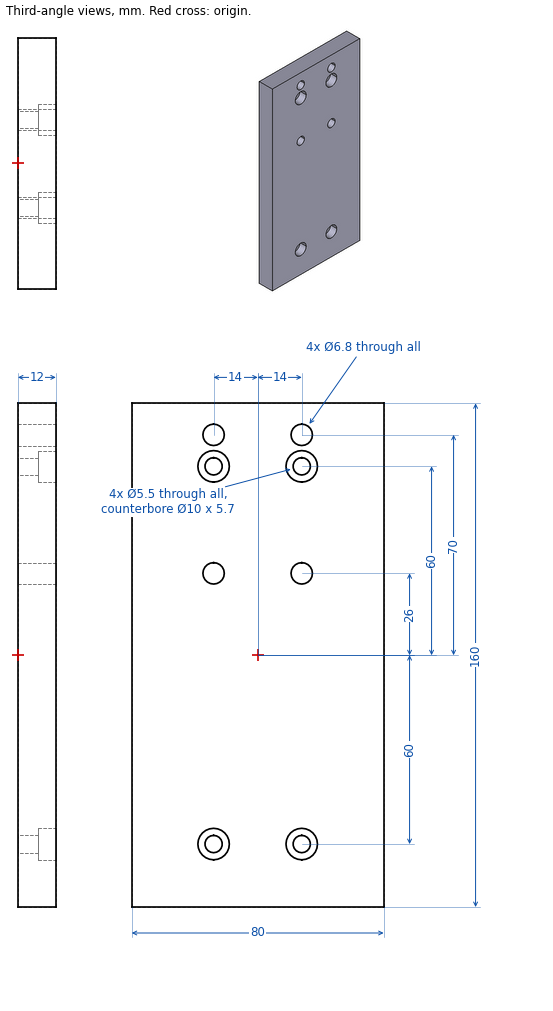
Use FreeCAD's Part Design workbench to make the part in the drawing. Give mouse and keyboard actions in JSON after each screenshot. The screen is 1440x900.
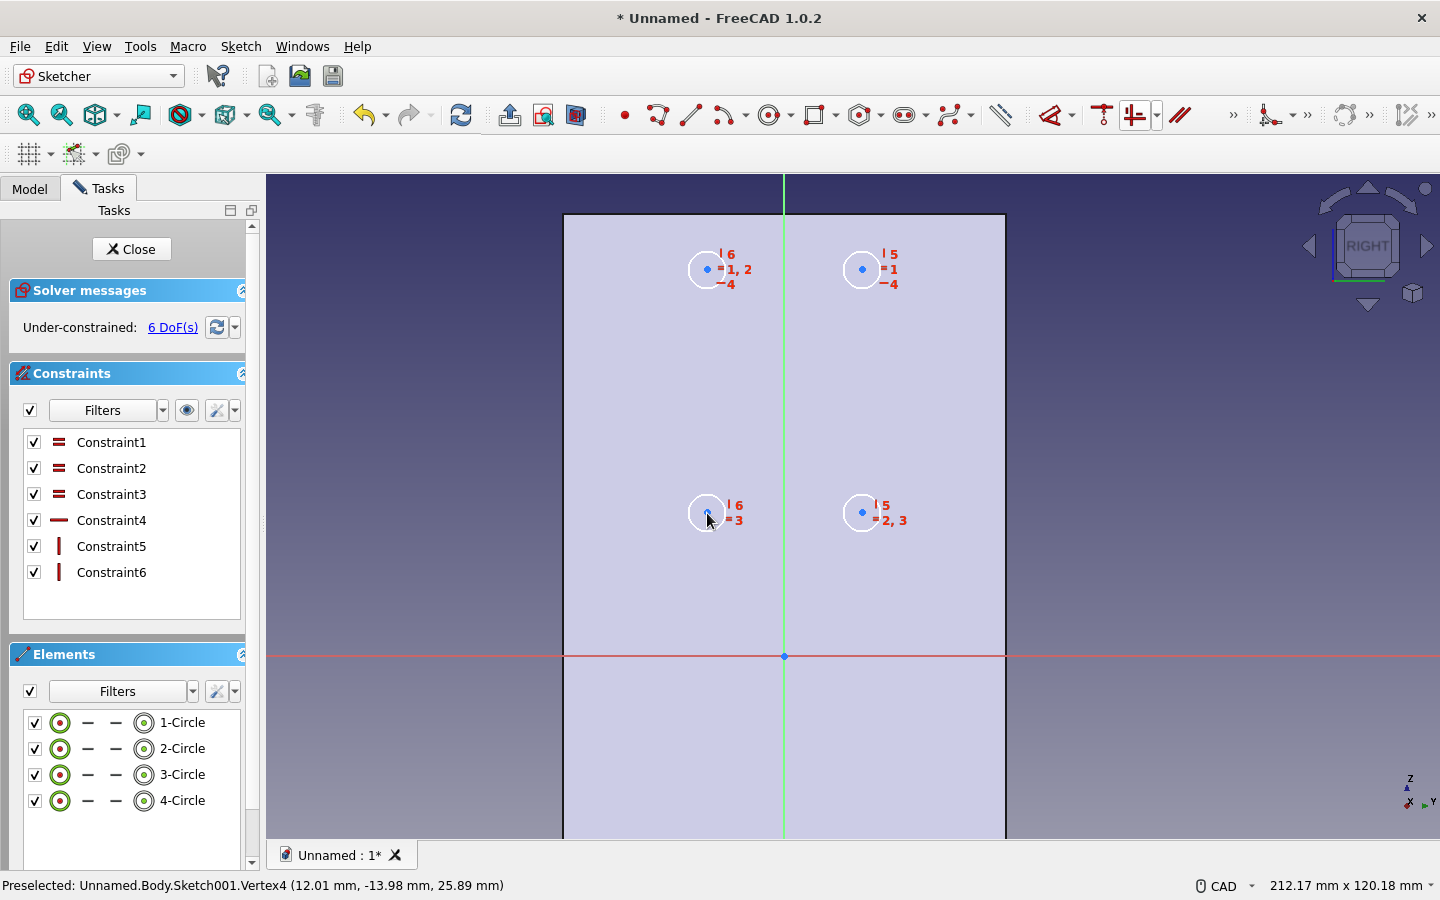
{"action": "left_click", "coordinate": [862, 513]}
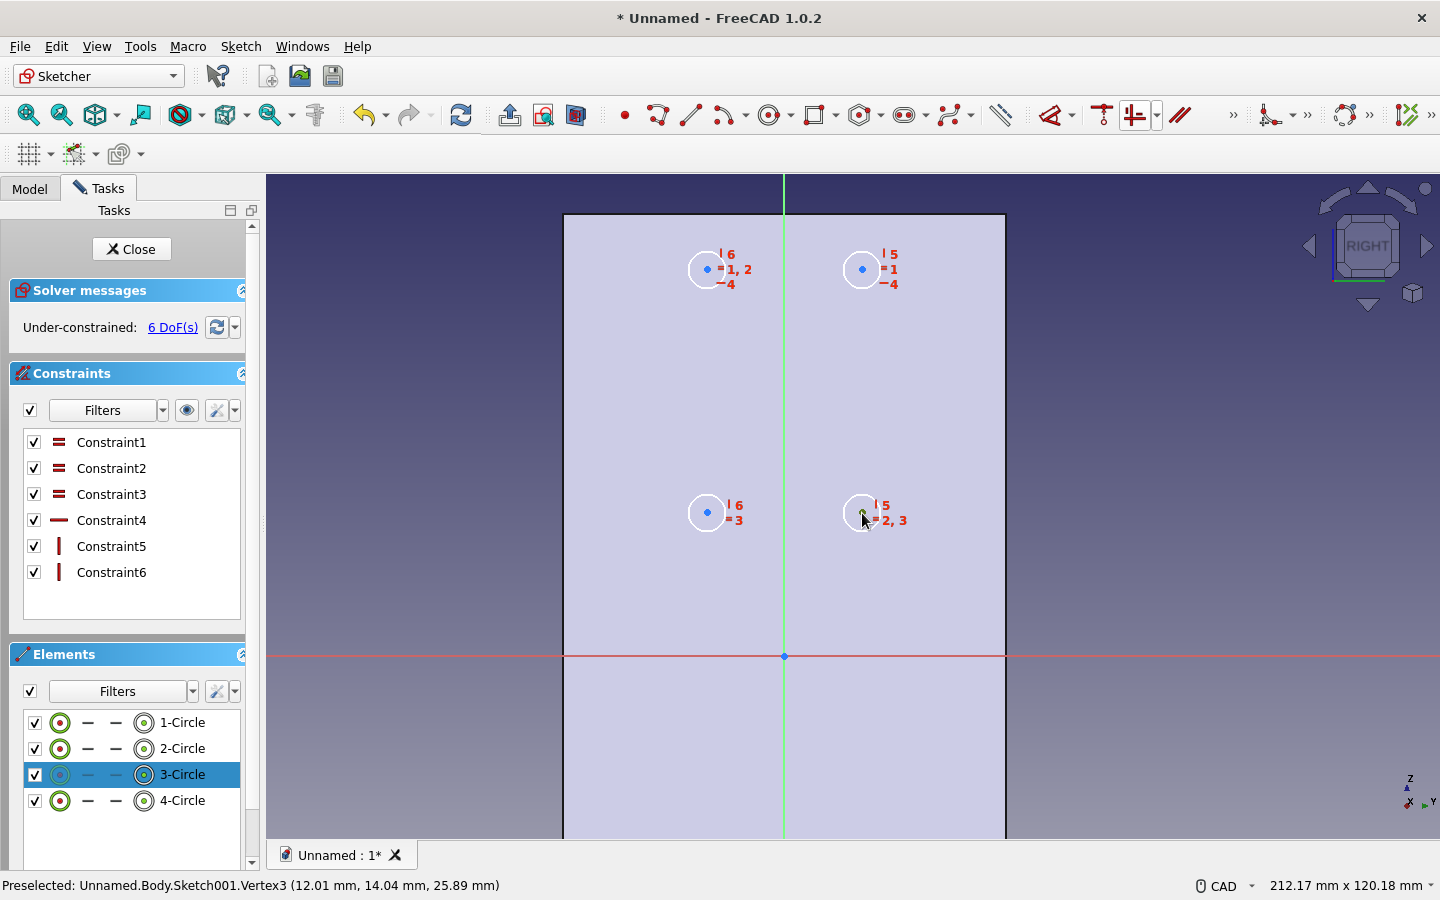
{"action": "left_click", "coordinate": [707, 513]}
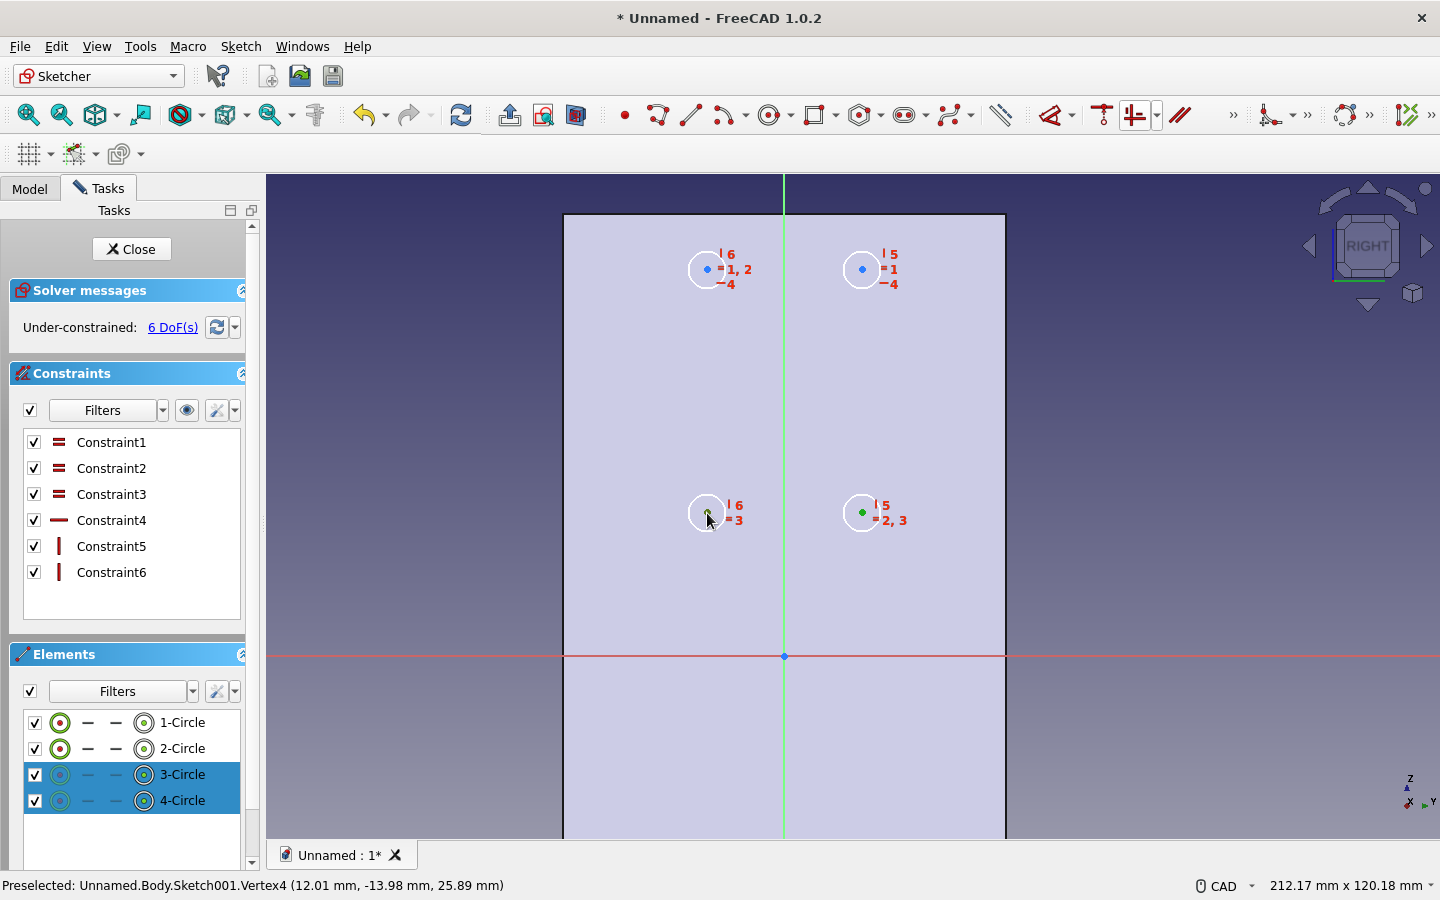
{"action": "key", "text": "h"}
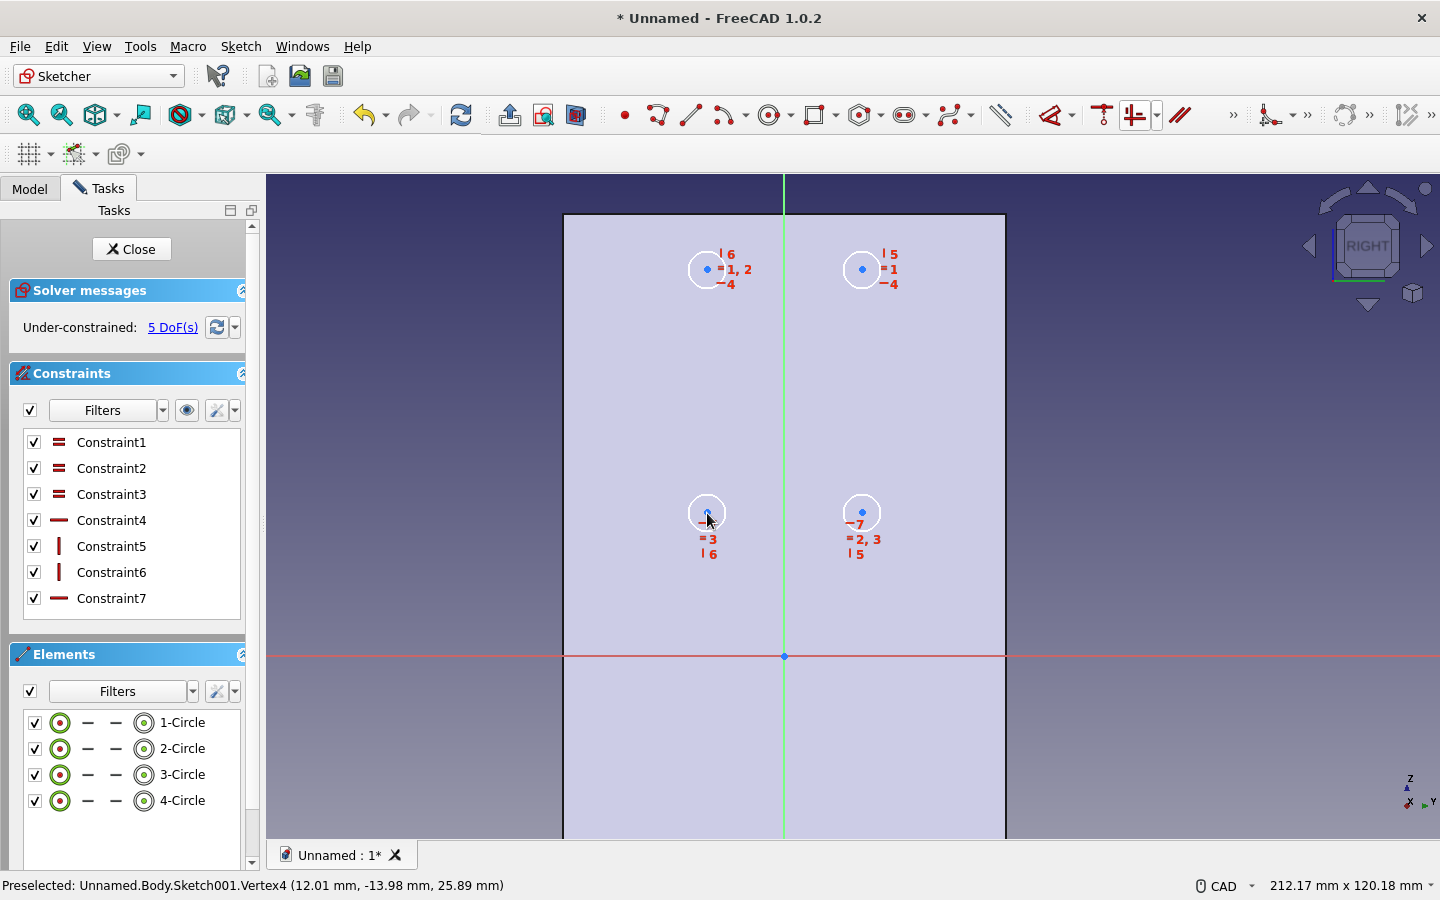
{"action": "left_click", "coordinate": [1050, 116]}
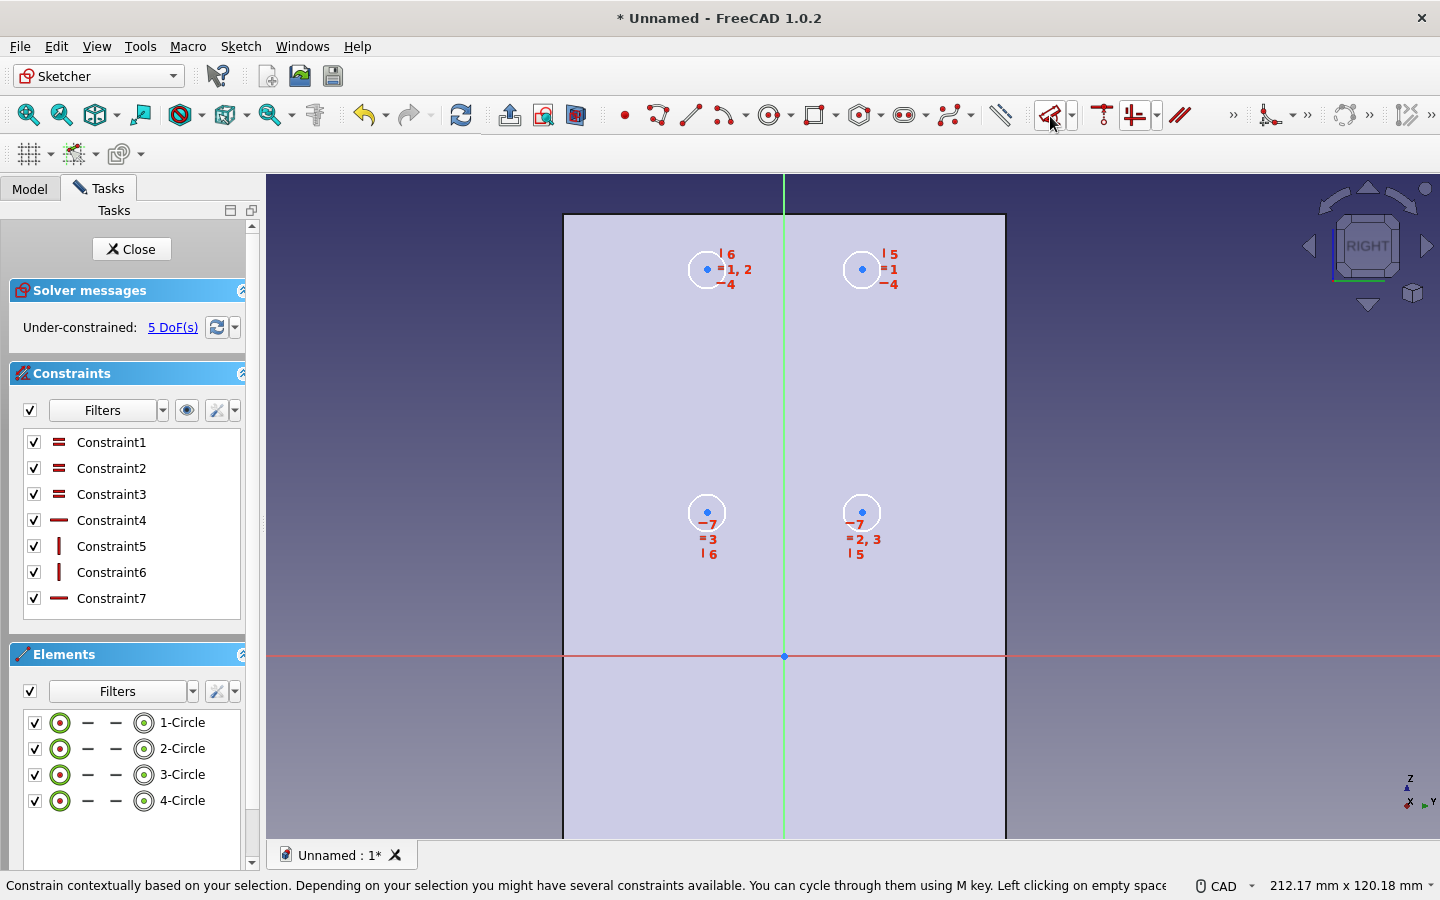
{"action": "left_click", "coordinate": [875, 257]}
{"action": "left_click", "coordinate": [898, 234]}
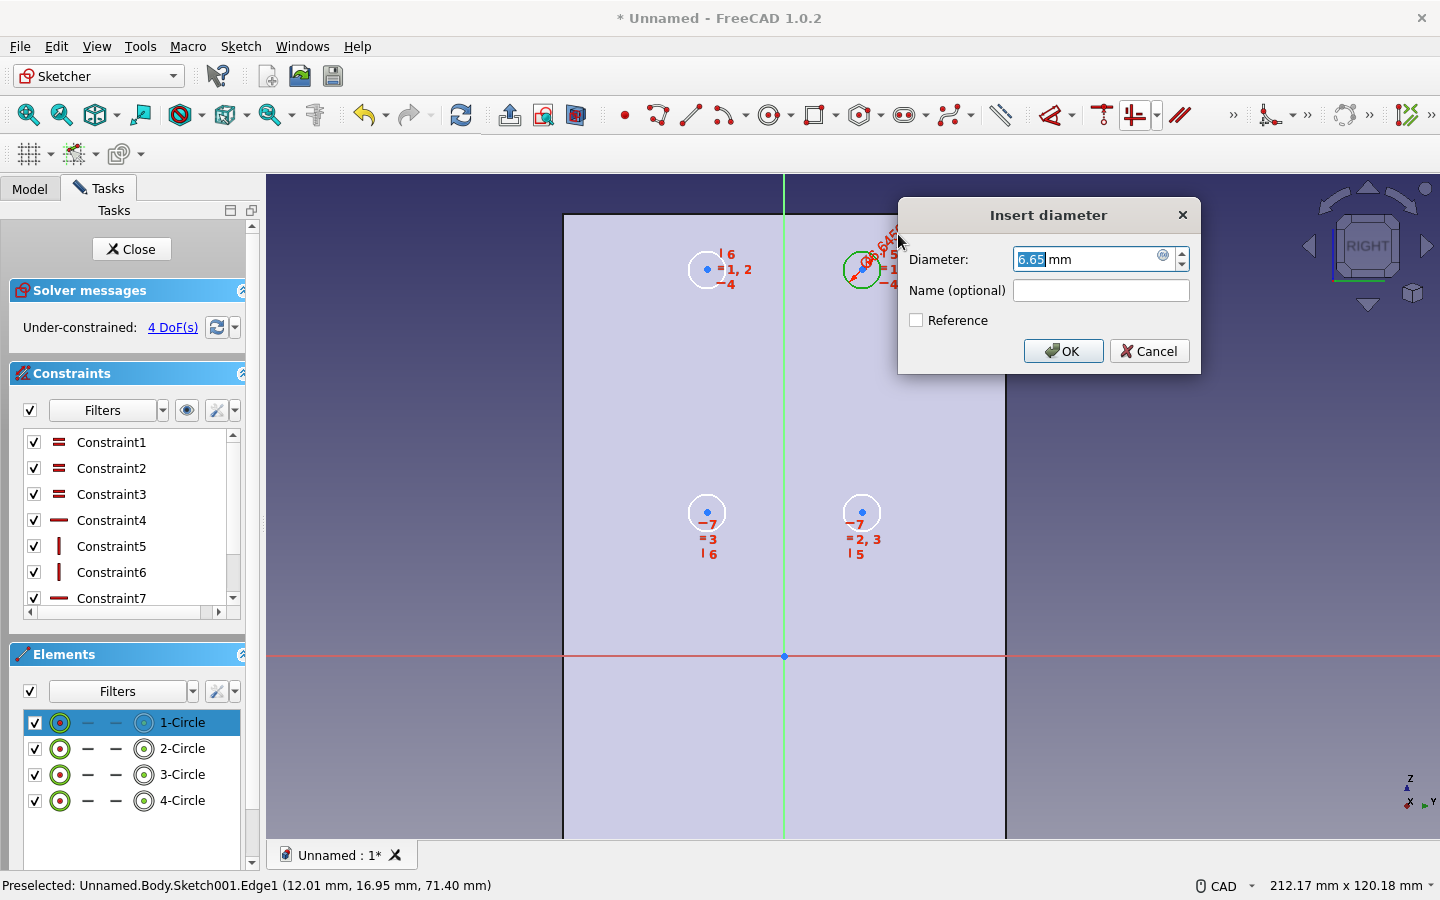
{"action": "type", "text": "6.8"}
{"action": "key", "text": "Return"}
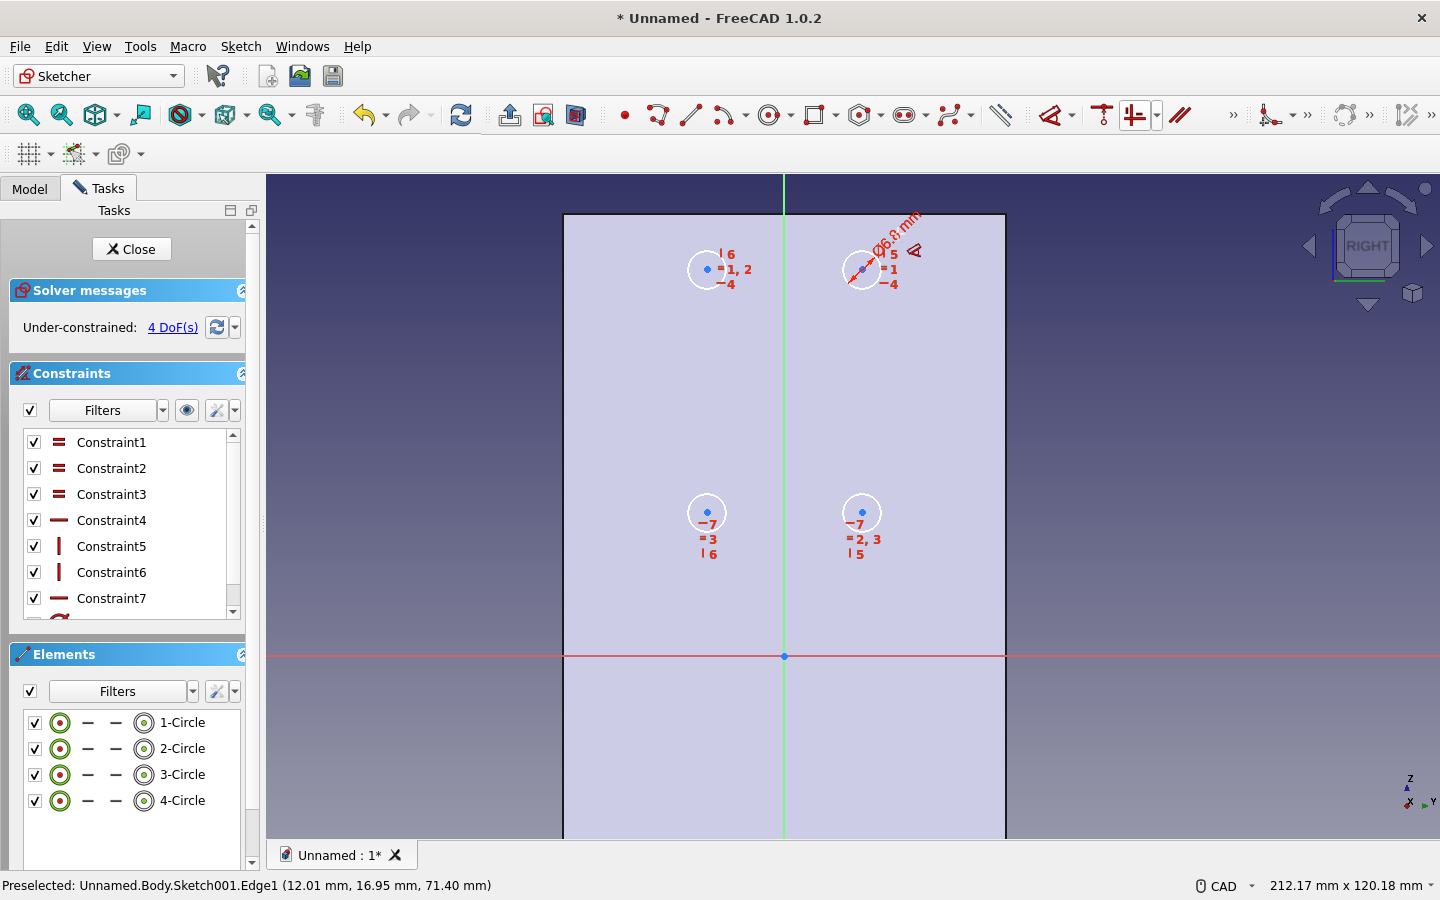
{"action": "left_click", "coordinate": [862, 270]}
{"action": "left_click", "coordinate": [823, 690]}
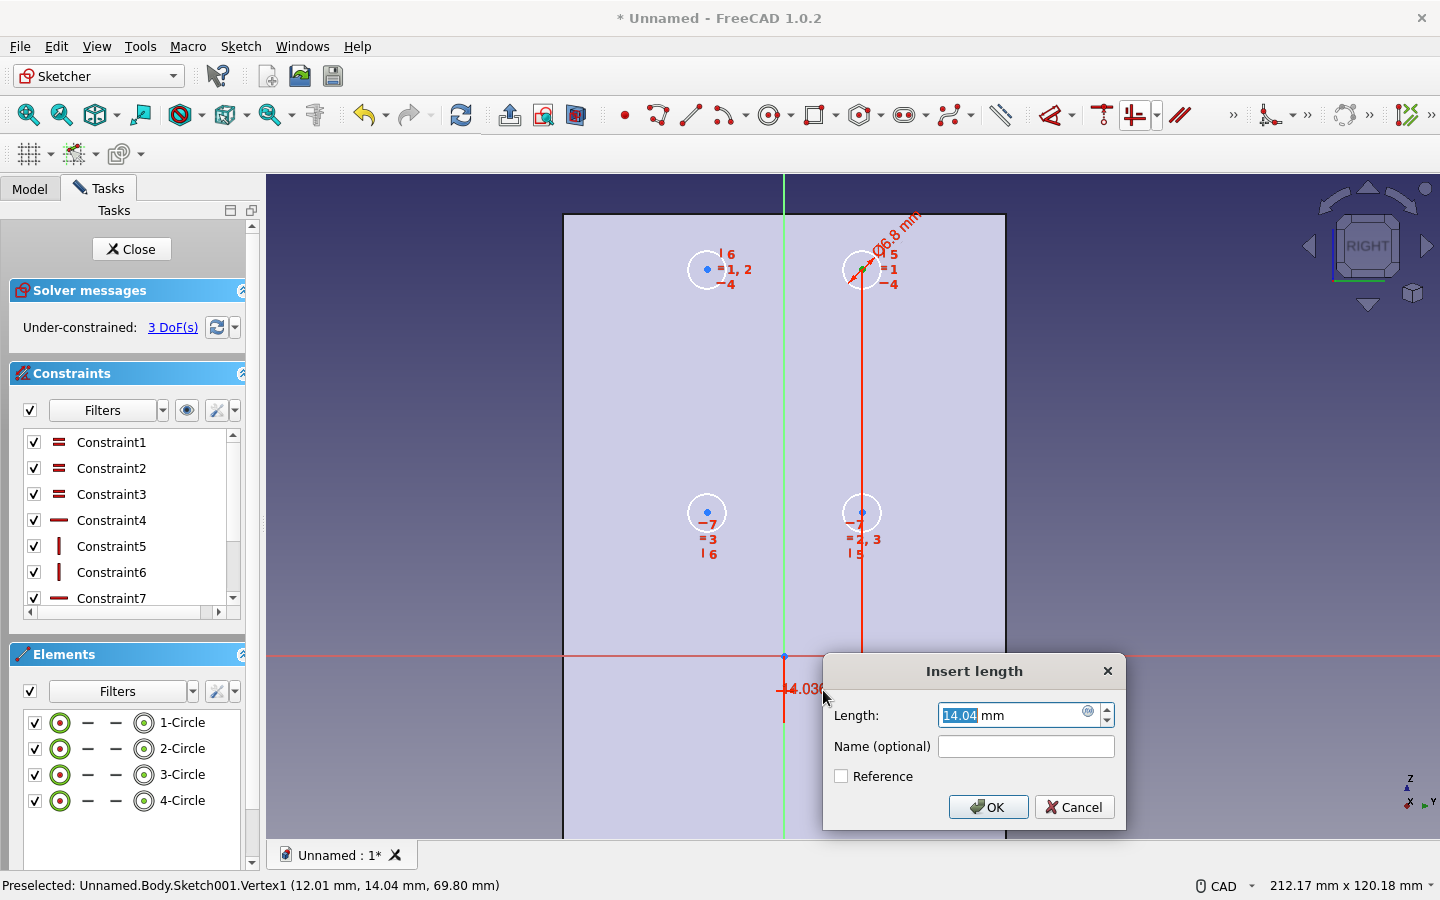
{"action": "type", "text": "14"}
{"action": "key", "text": "Return"}